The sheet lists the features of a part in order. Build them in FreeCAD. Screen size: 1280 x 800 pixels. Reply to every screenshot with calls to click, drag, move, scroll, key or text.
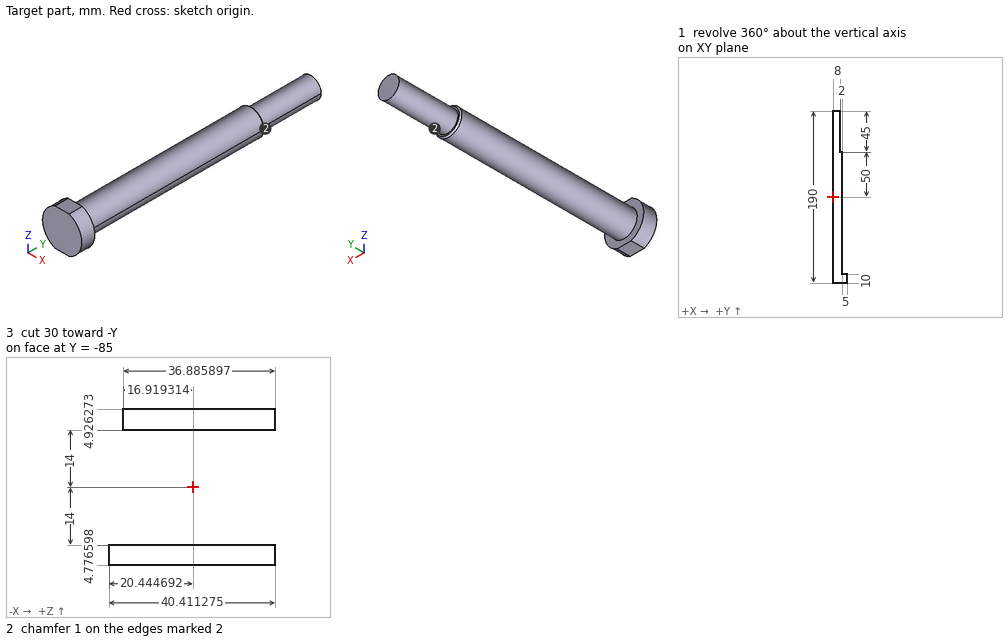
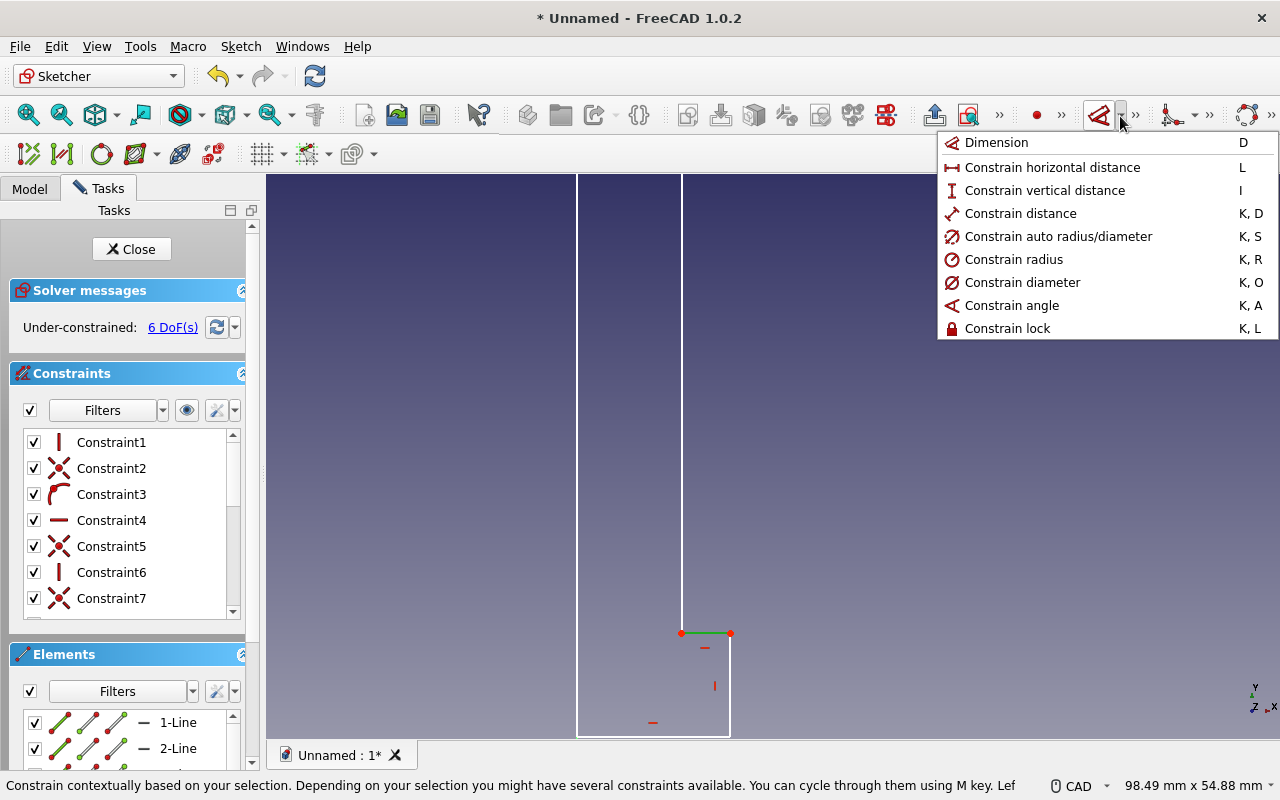
click(1108, 168)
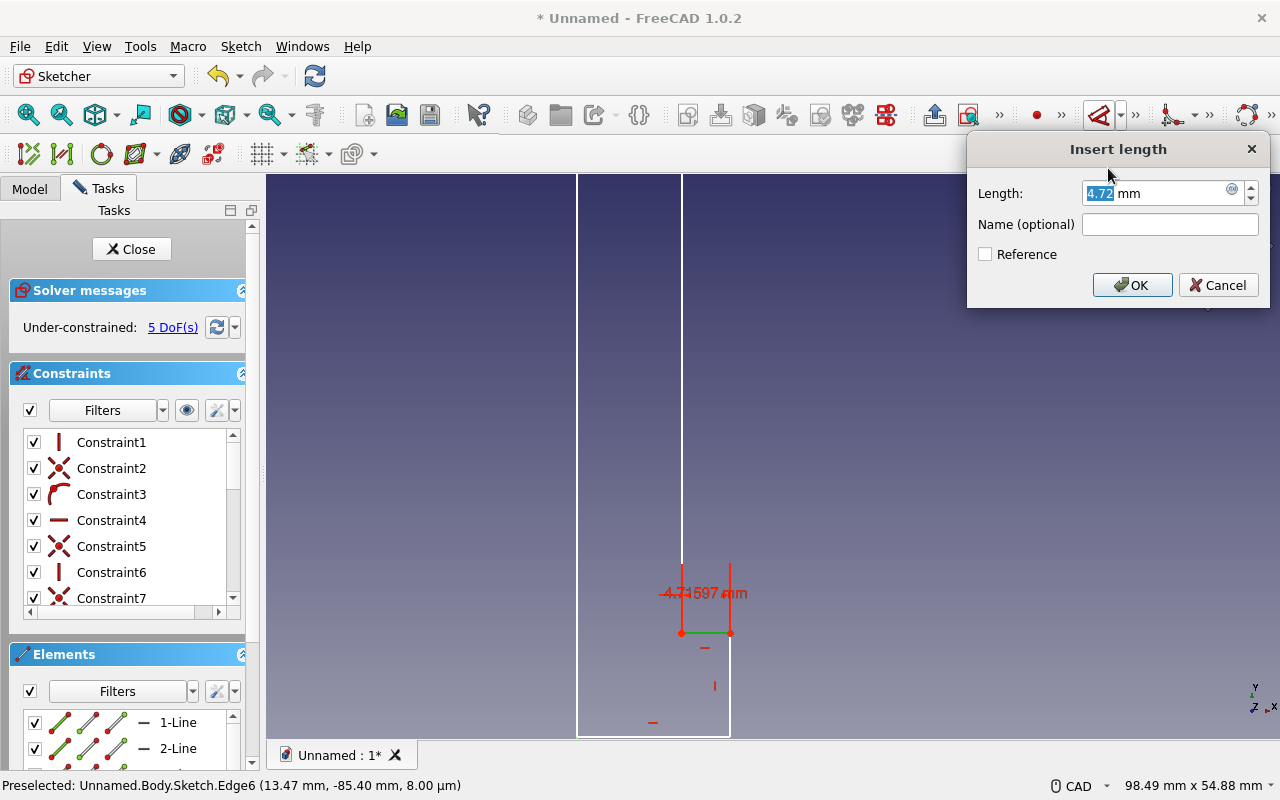
text(5)
key(Return)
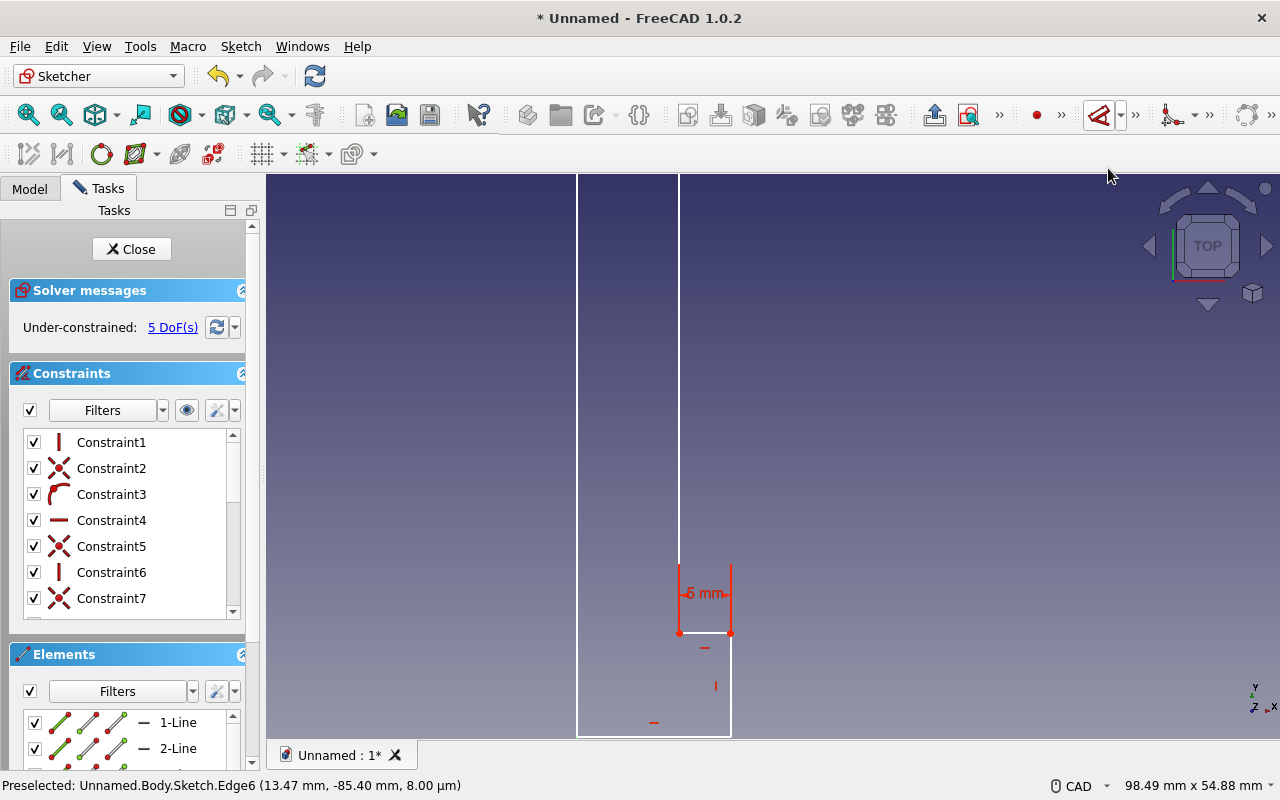
scroll(717, 634, down, 8)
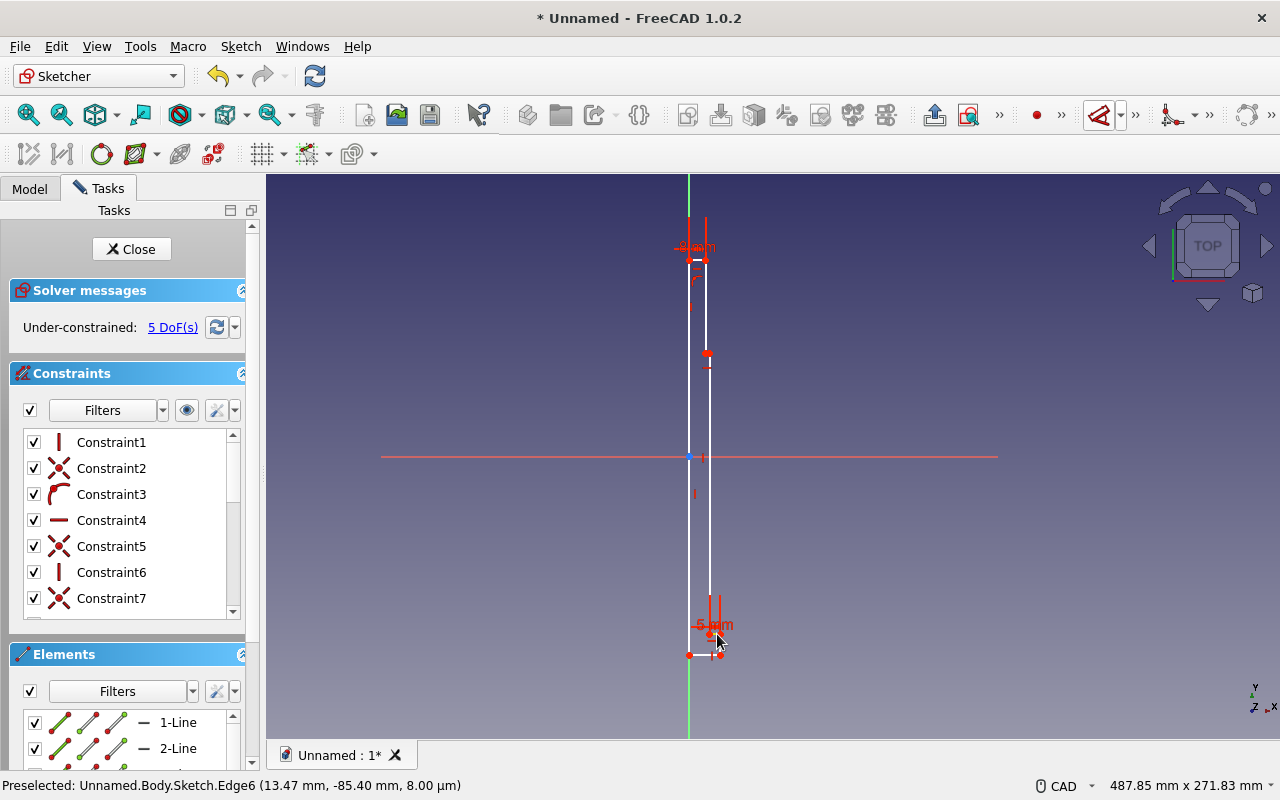
scroll(708, 353, up, 12)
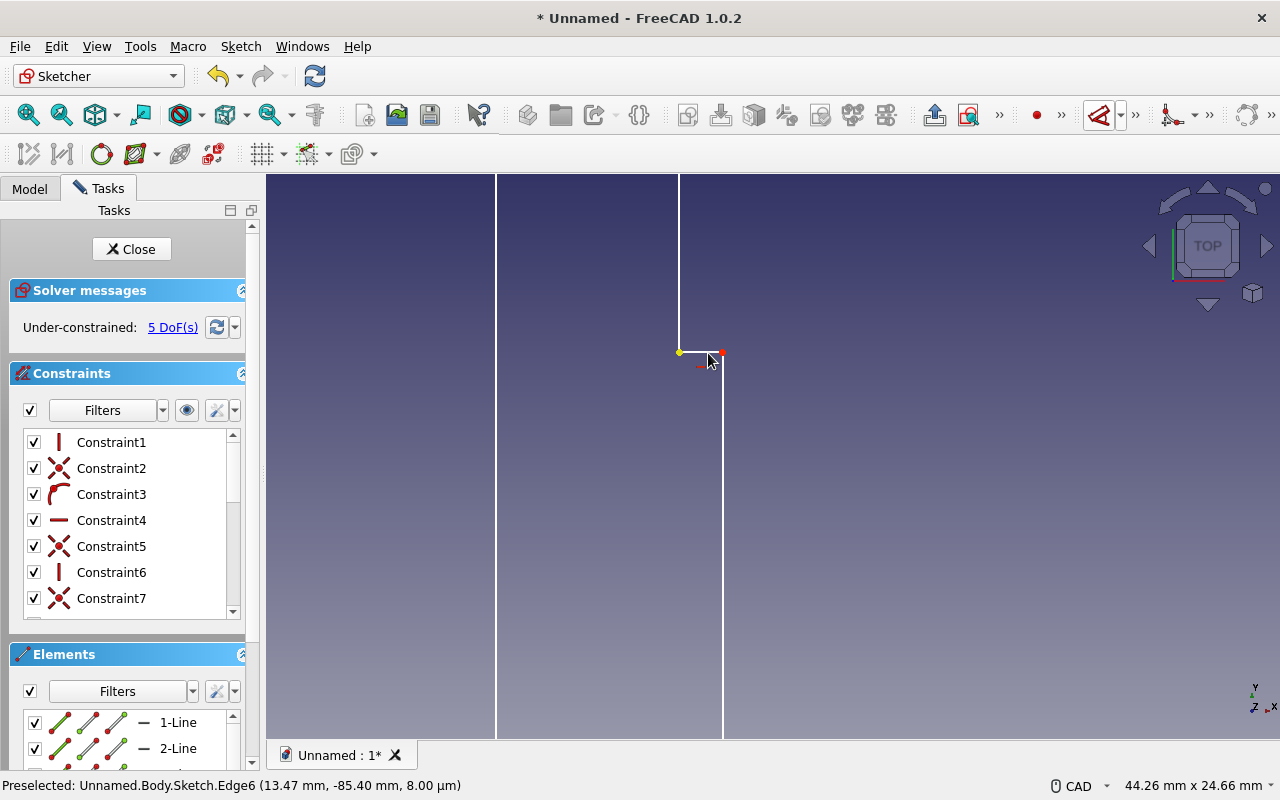
click(701, 352)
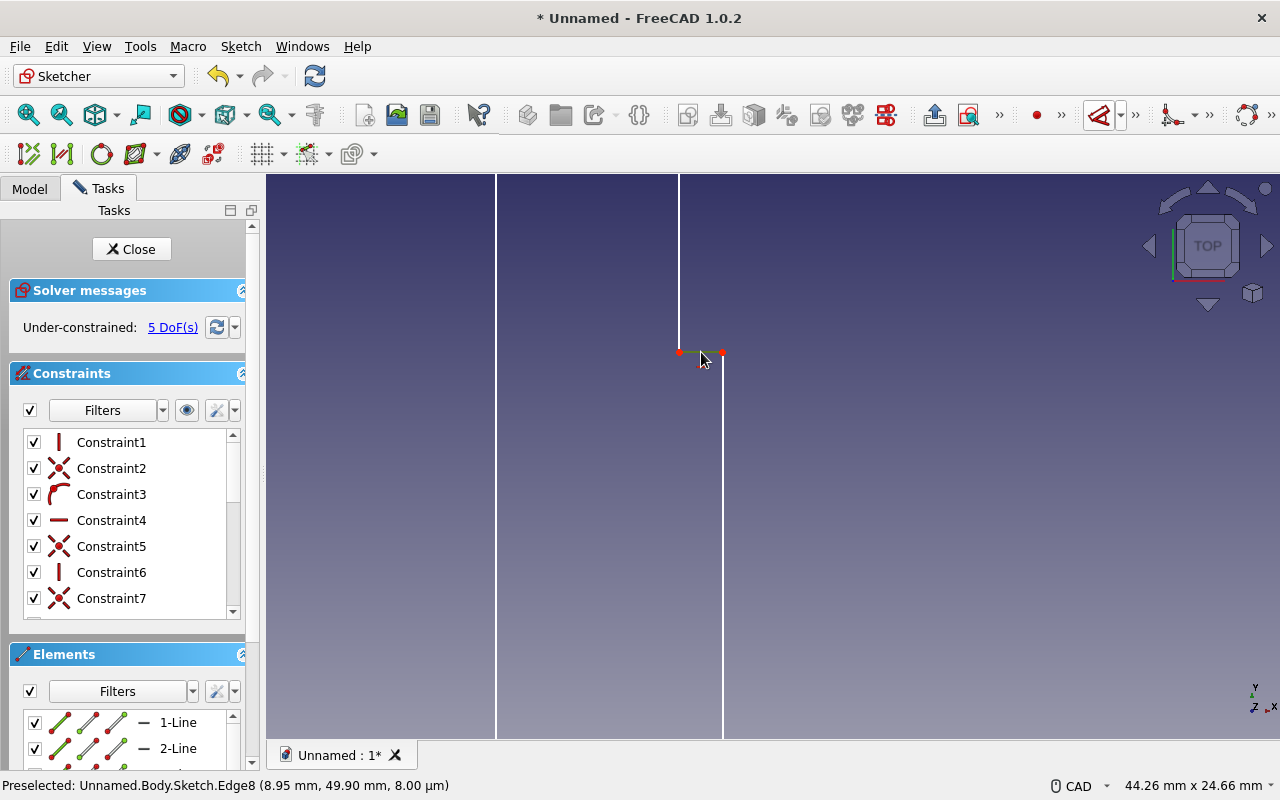
key(l)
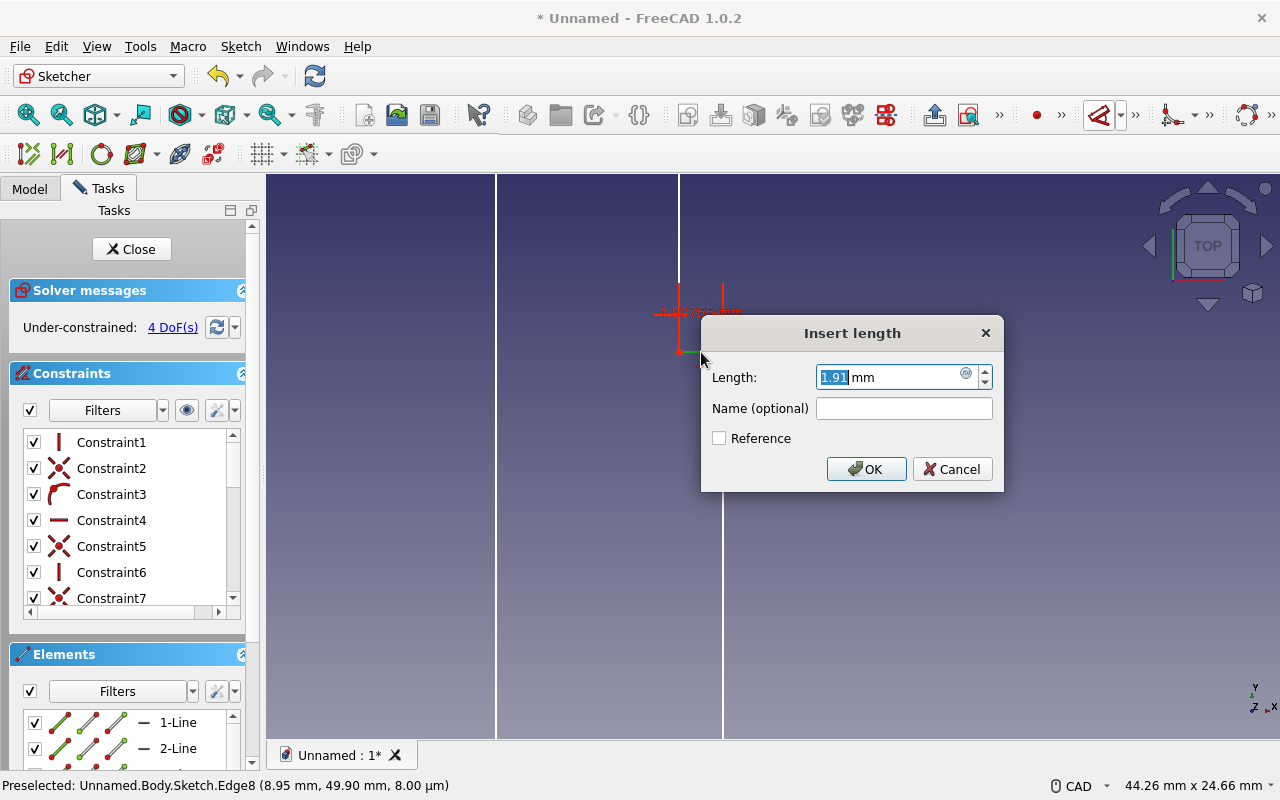
text(2)
key(Return)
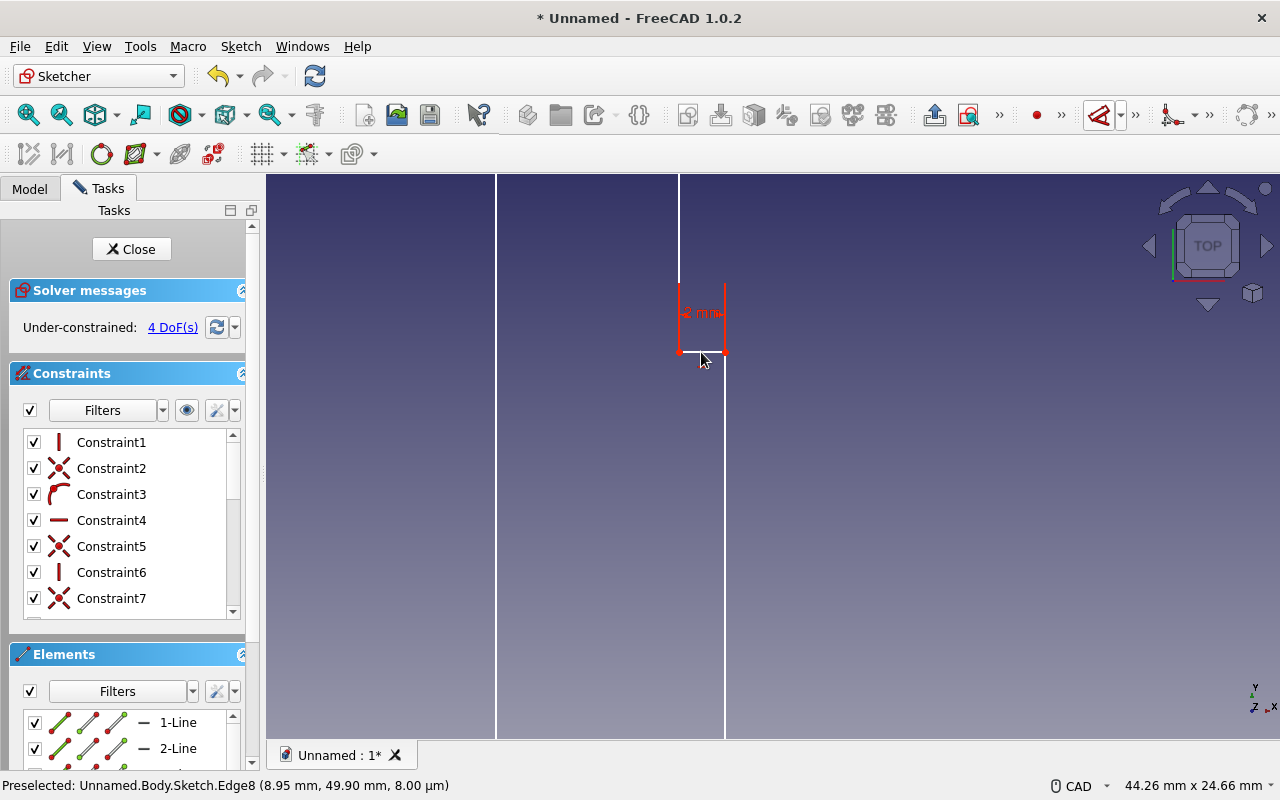
scroll(708, 353, down, 12)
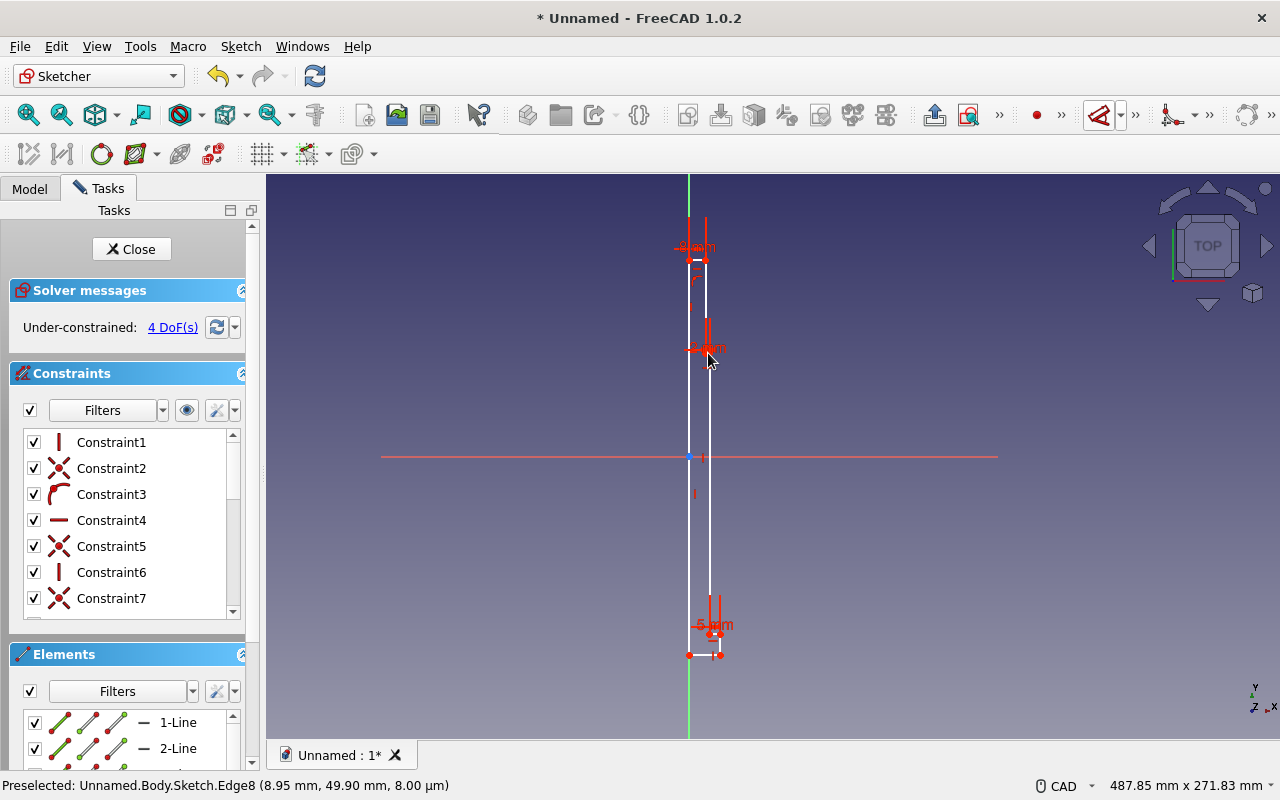
click(706, 325)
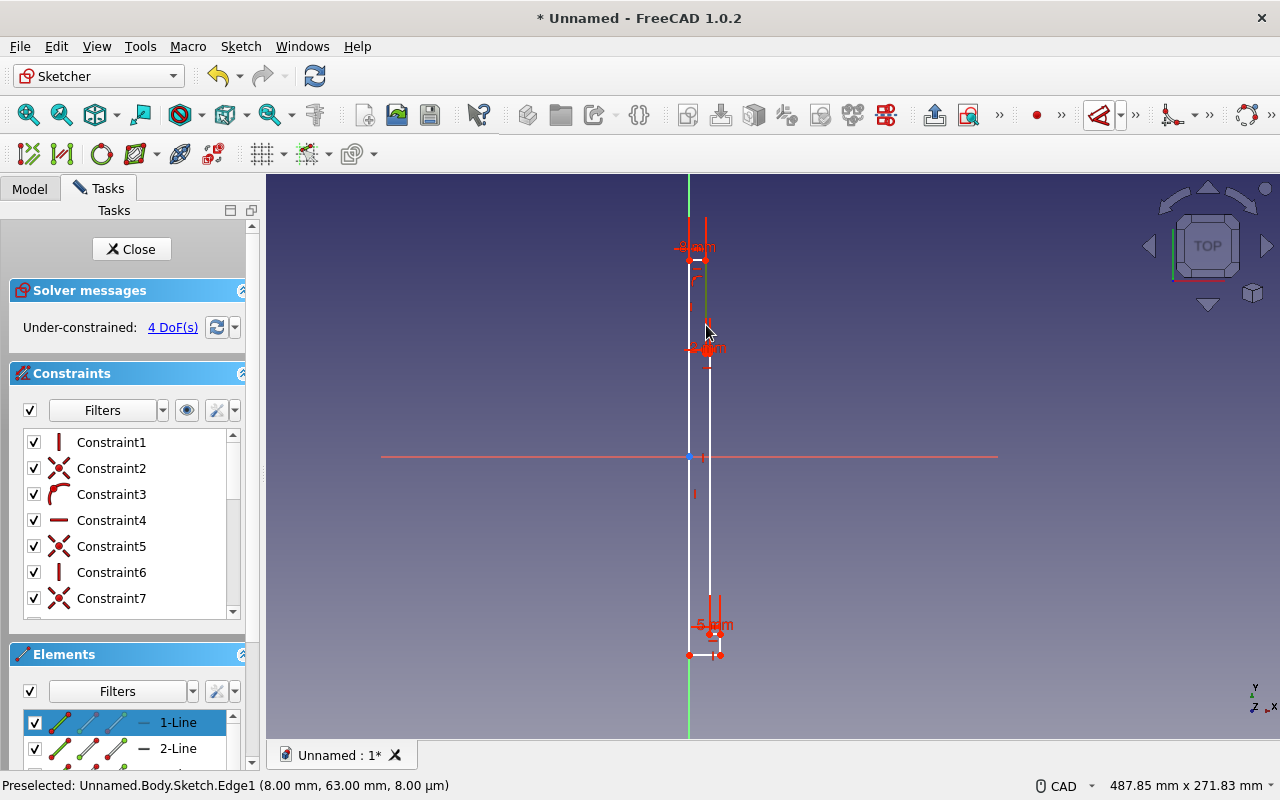
key(i)